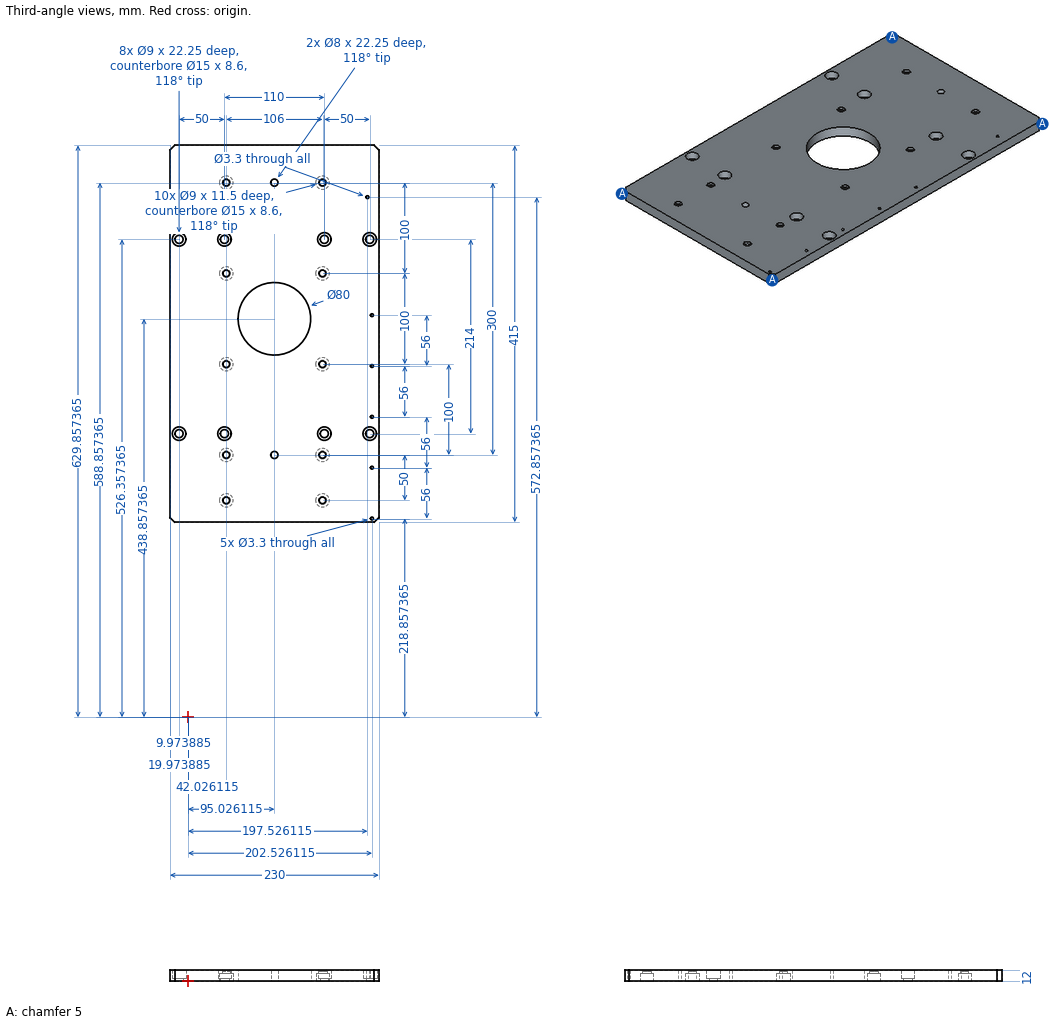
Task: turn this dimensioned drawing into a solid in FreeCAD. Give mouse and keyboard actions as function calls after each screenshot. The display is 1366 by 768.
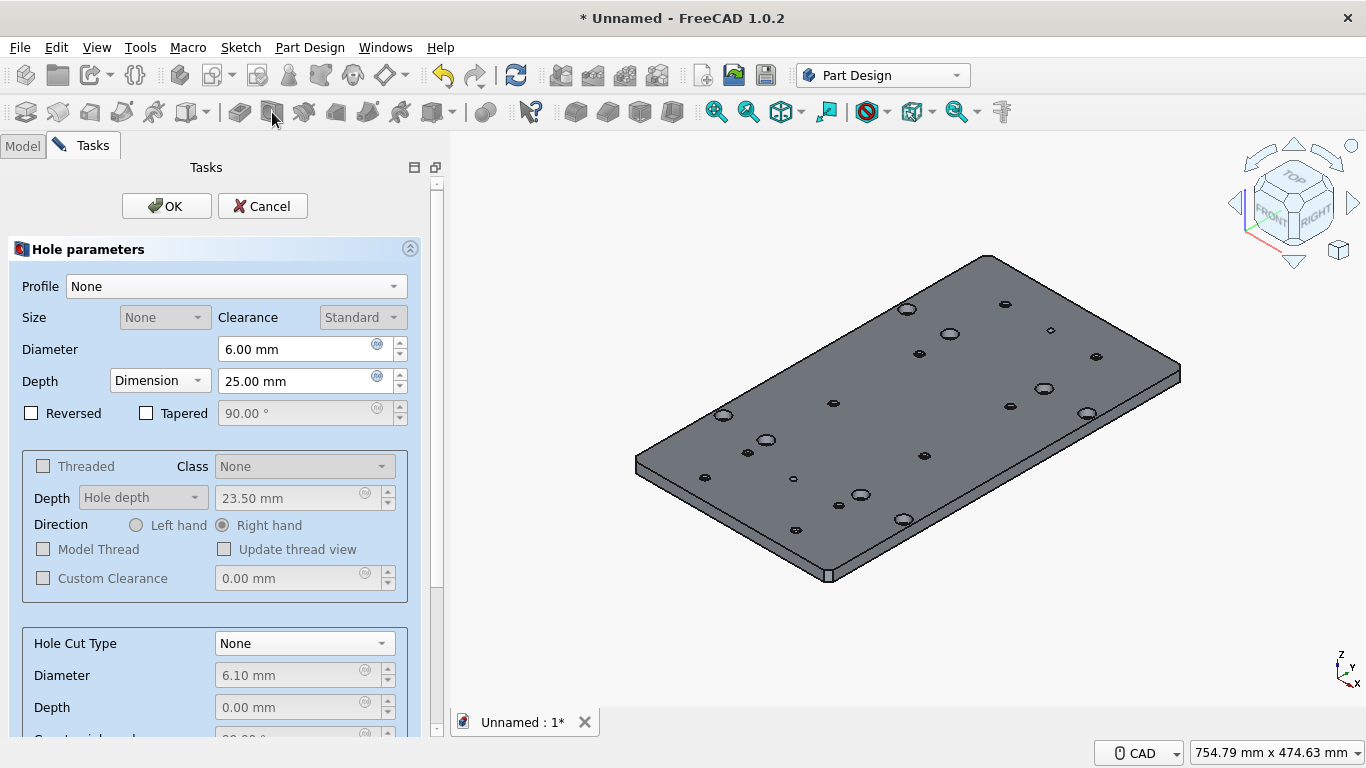
triple_click(305, 349)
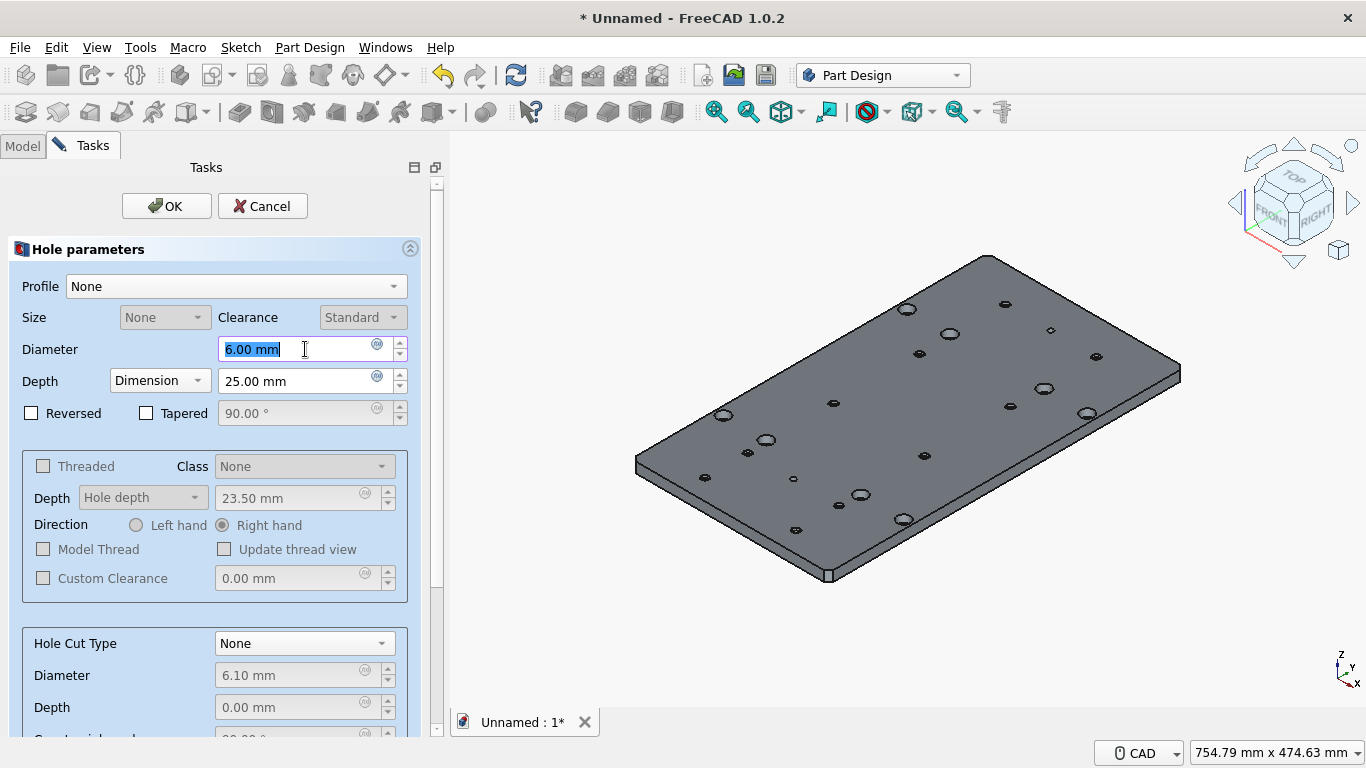
text(8)
key(Tab)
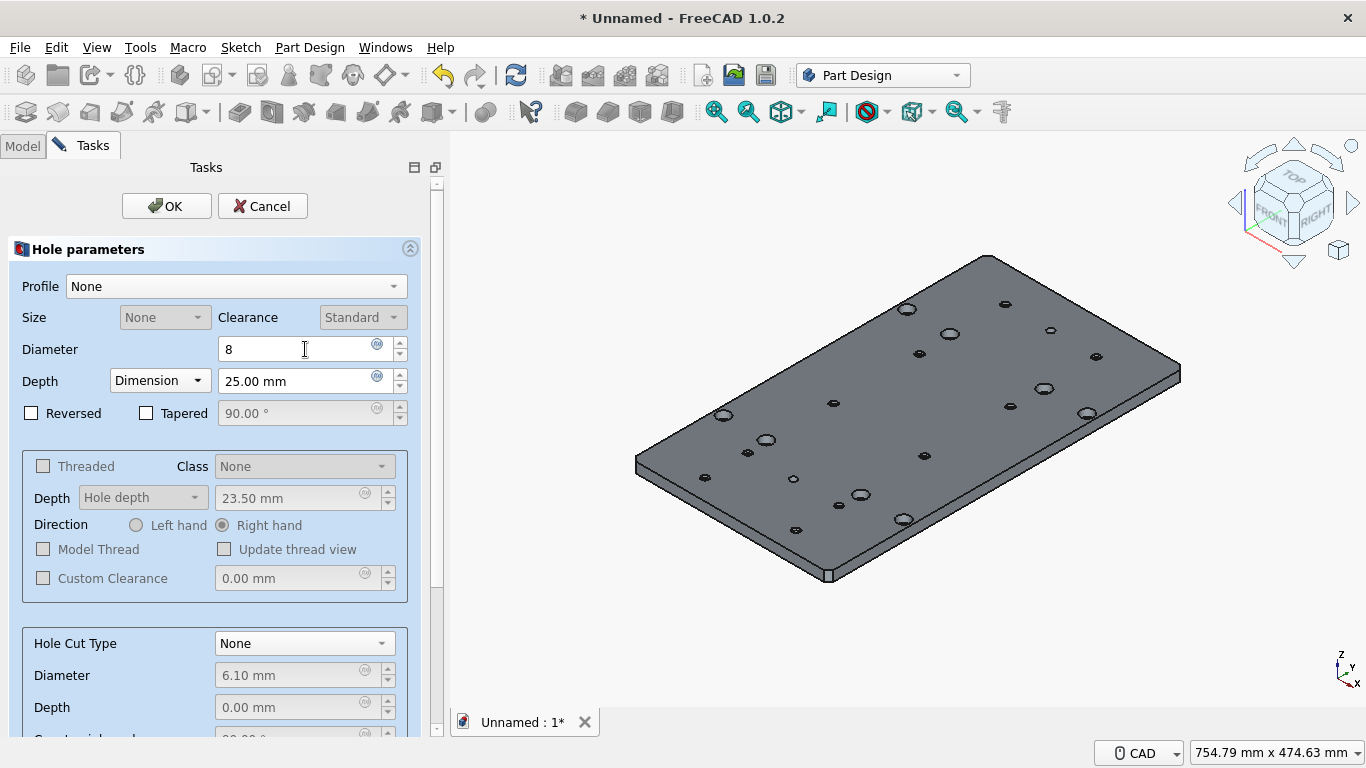
triple_click(305, 381)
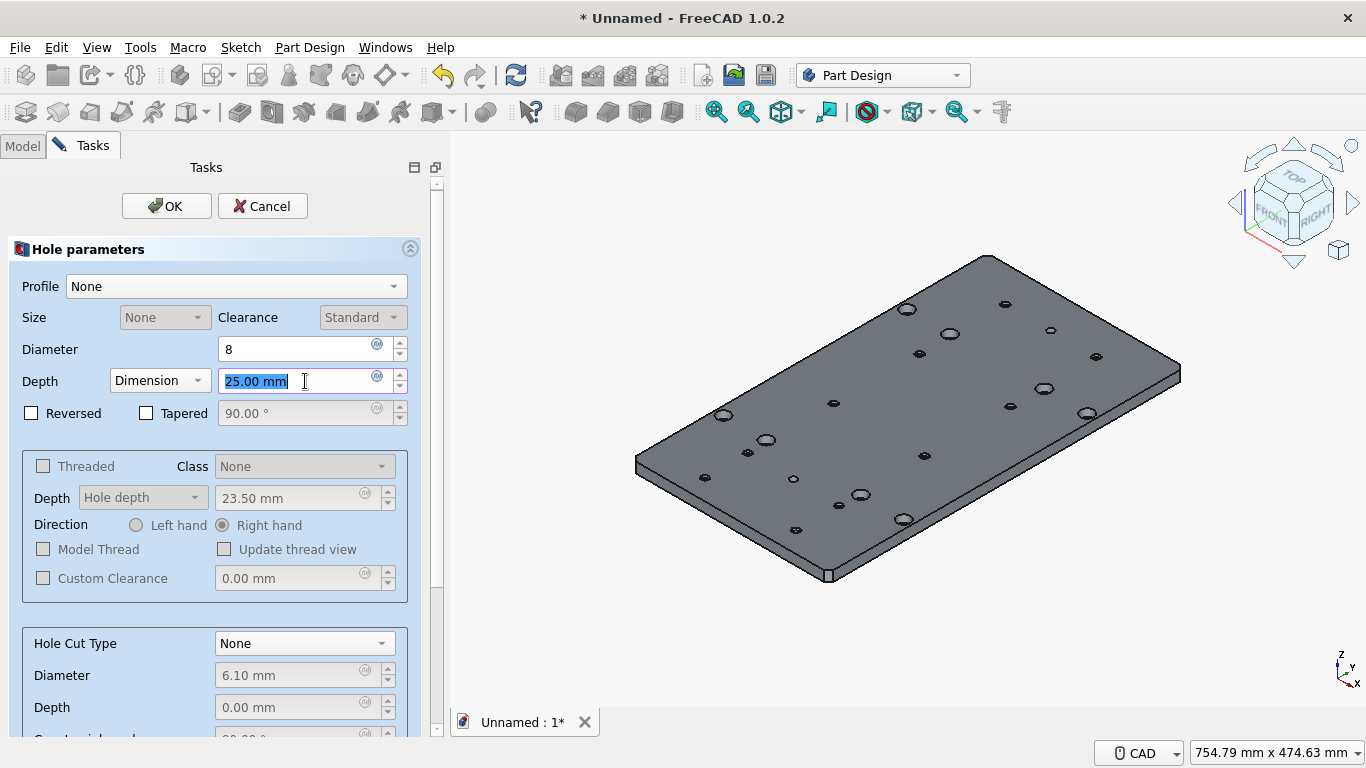
text(22.25)
key(Tab)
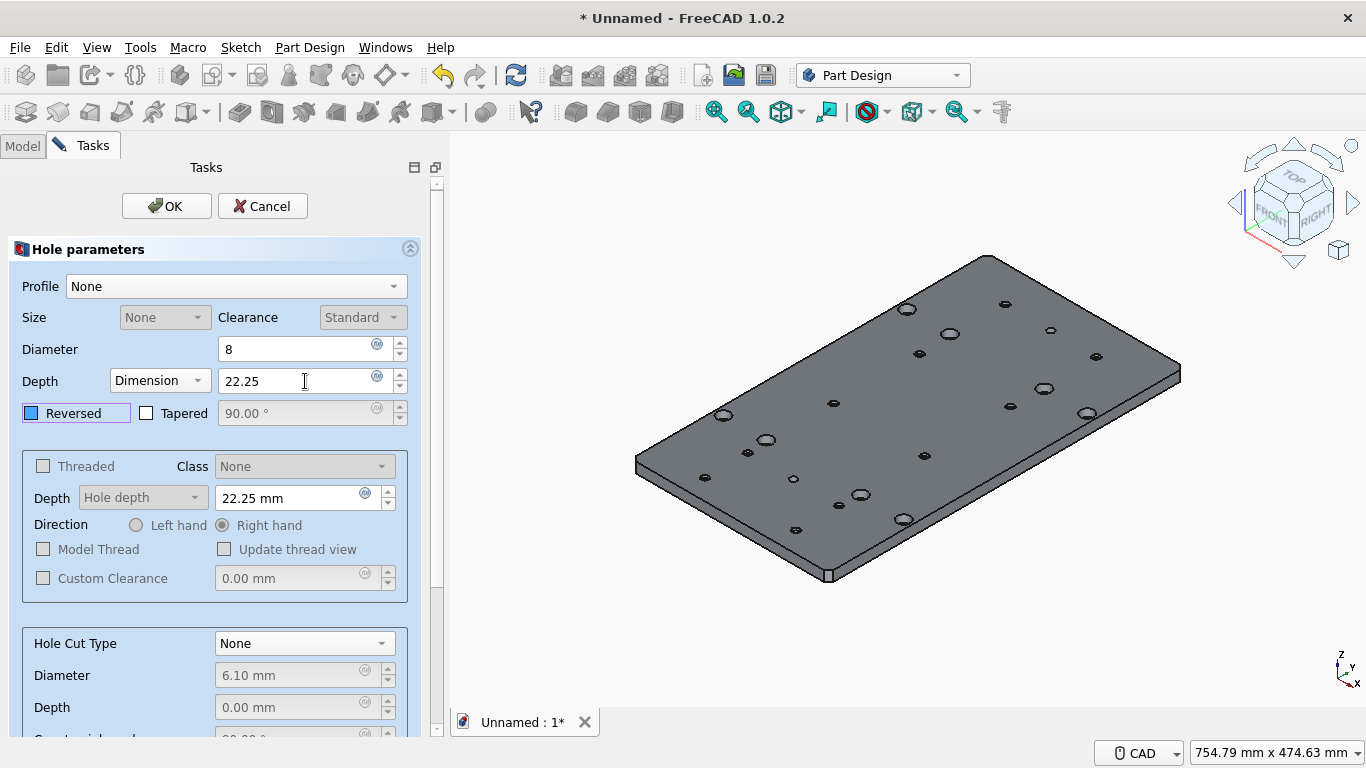
click(167, 206)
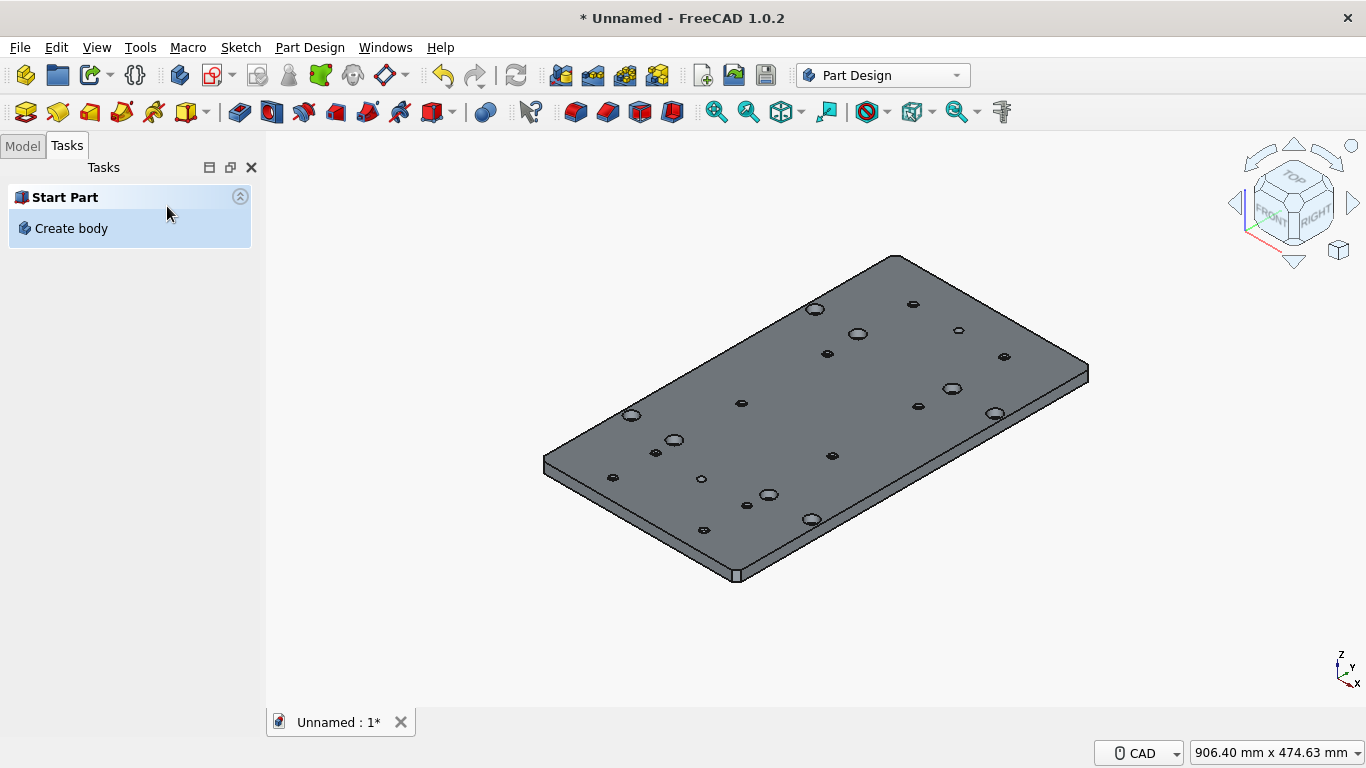
click(816, 412)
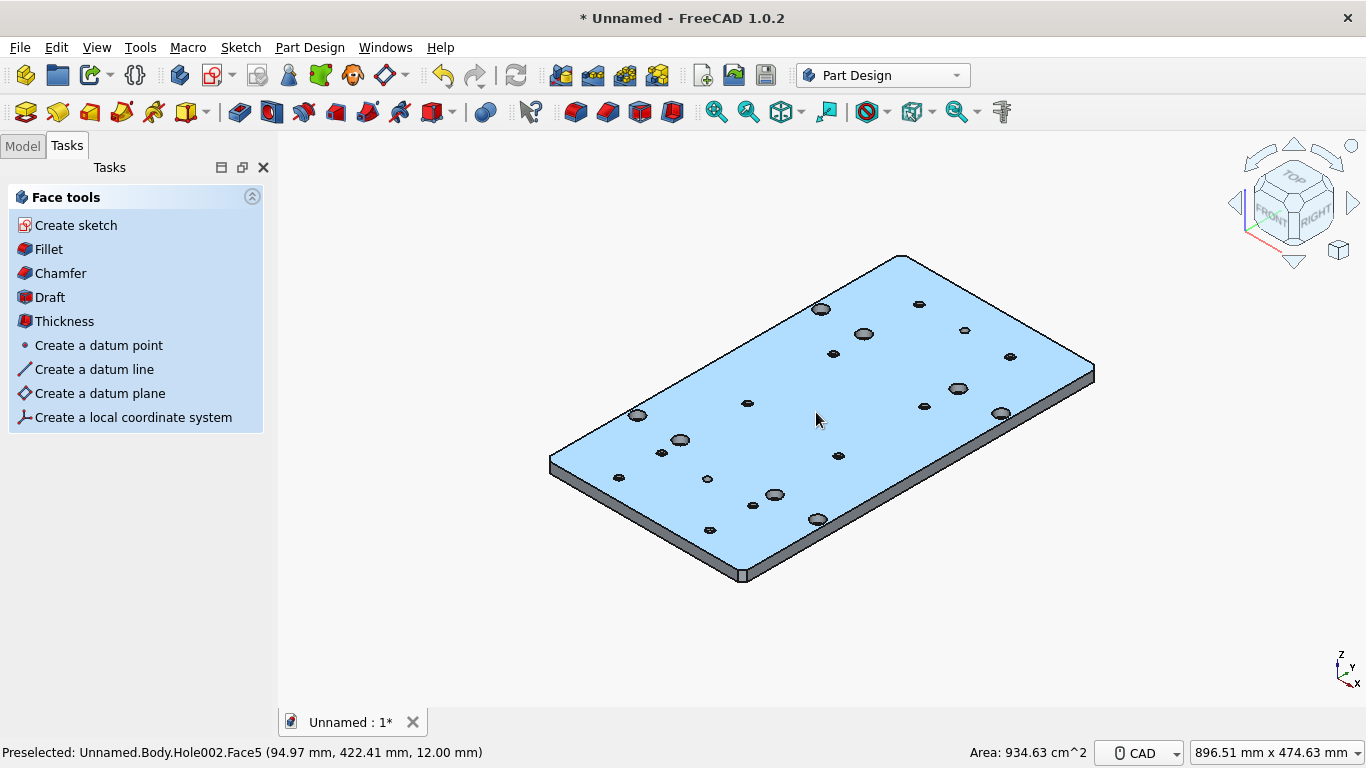
click(212, 76)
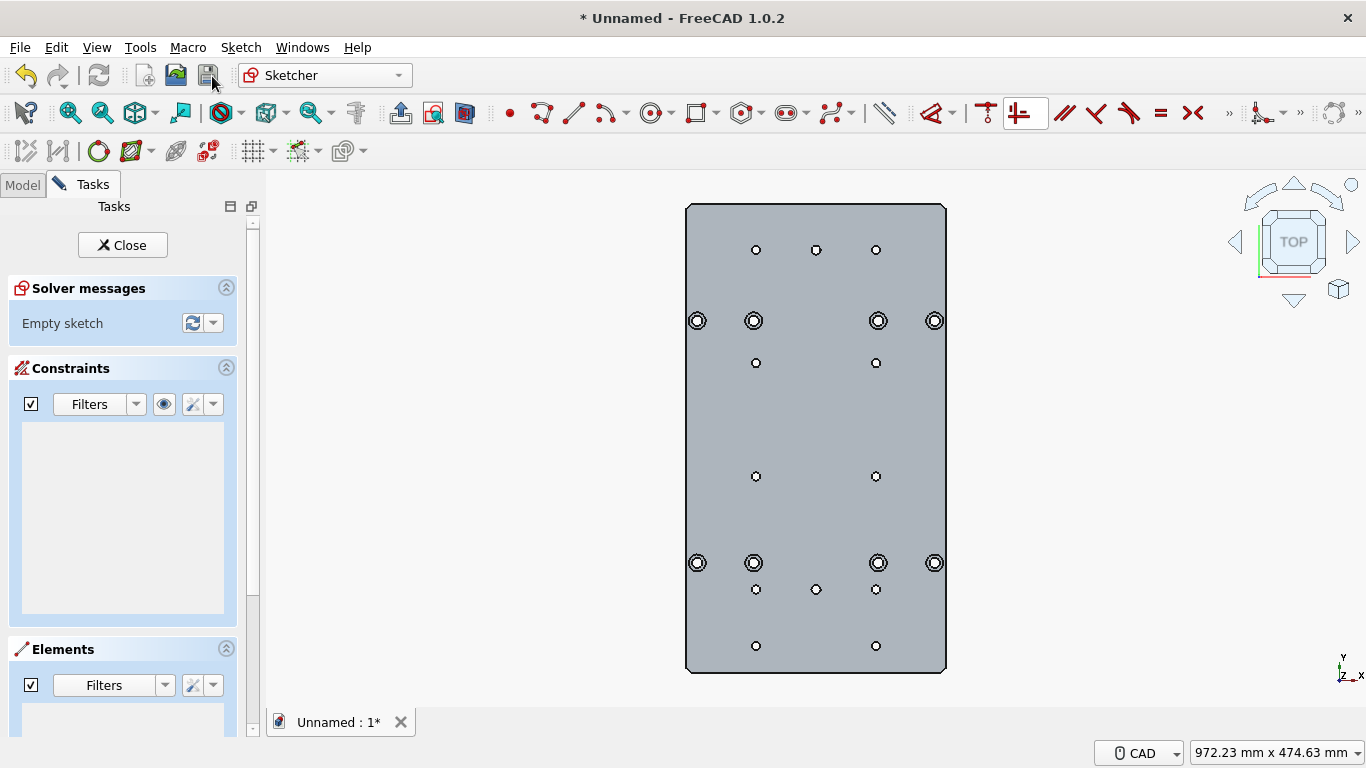
scroll(654, 198, down, 3)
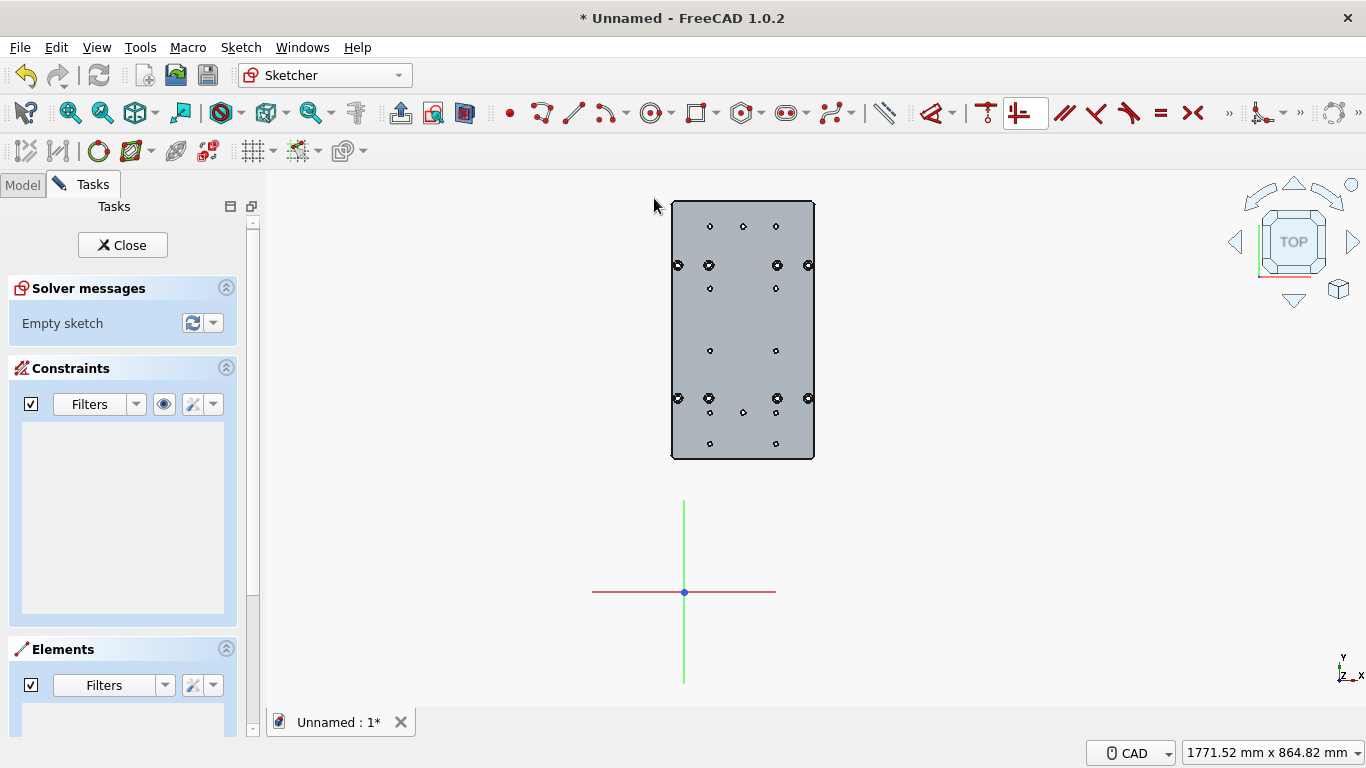
click(652, 114)